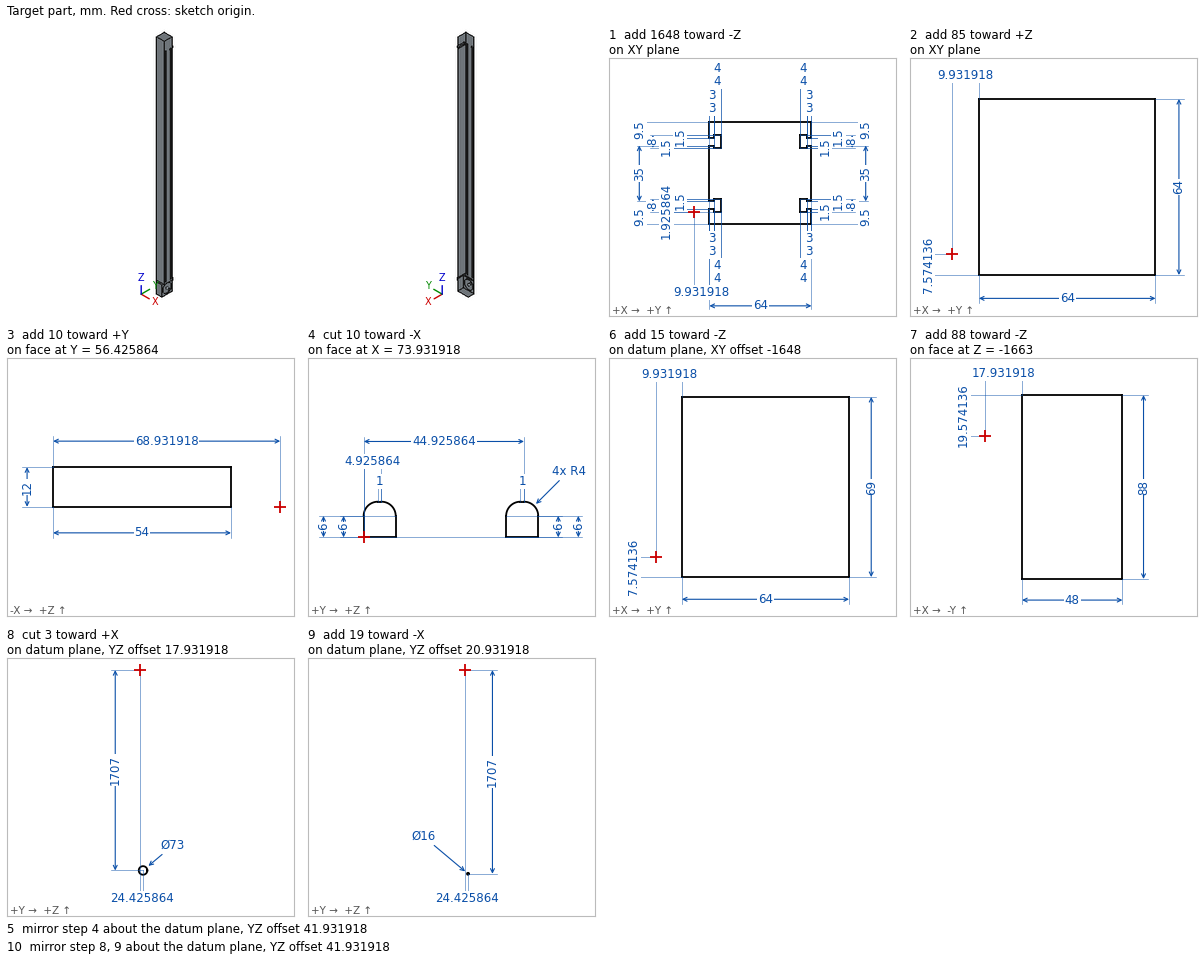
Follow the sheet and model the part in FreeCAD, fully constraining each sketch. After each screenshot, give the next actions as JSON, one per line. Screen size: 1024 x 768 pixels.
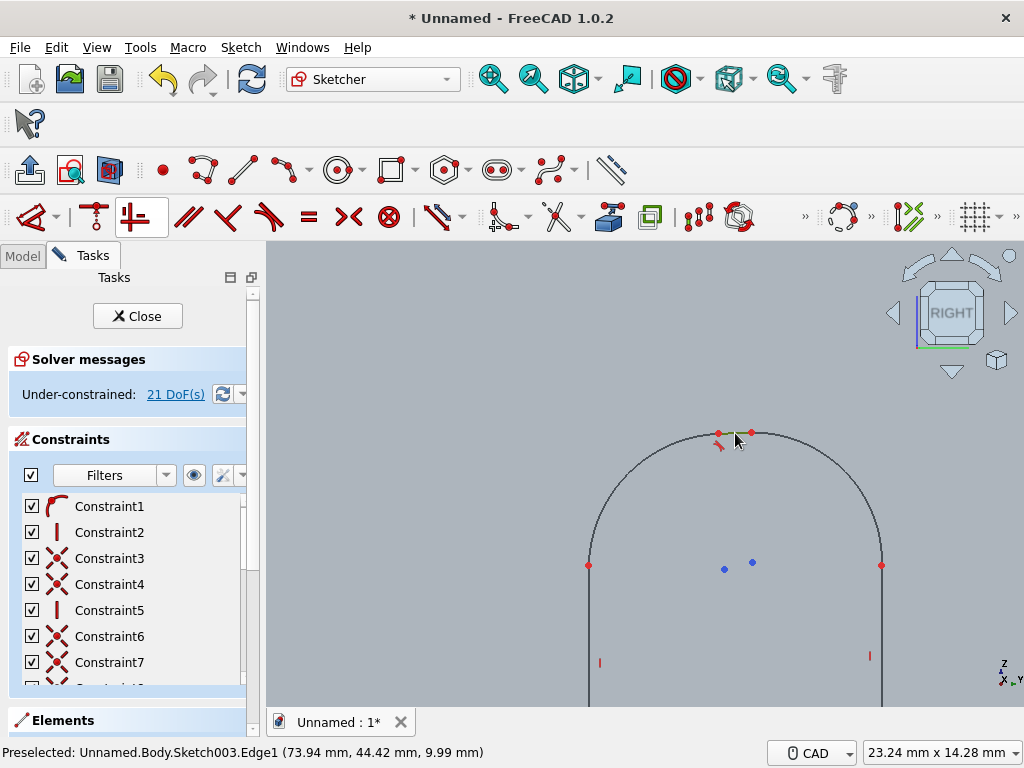
{"action": "scroll", "coordinate": [738, 434], "scroll_direction": "down", "scroll_amount": 7}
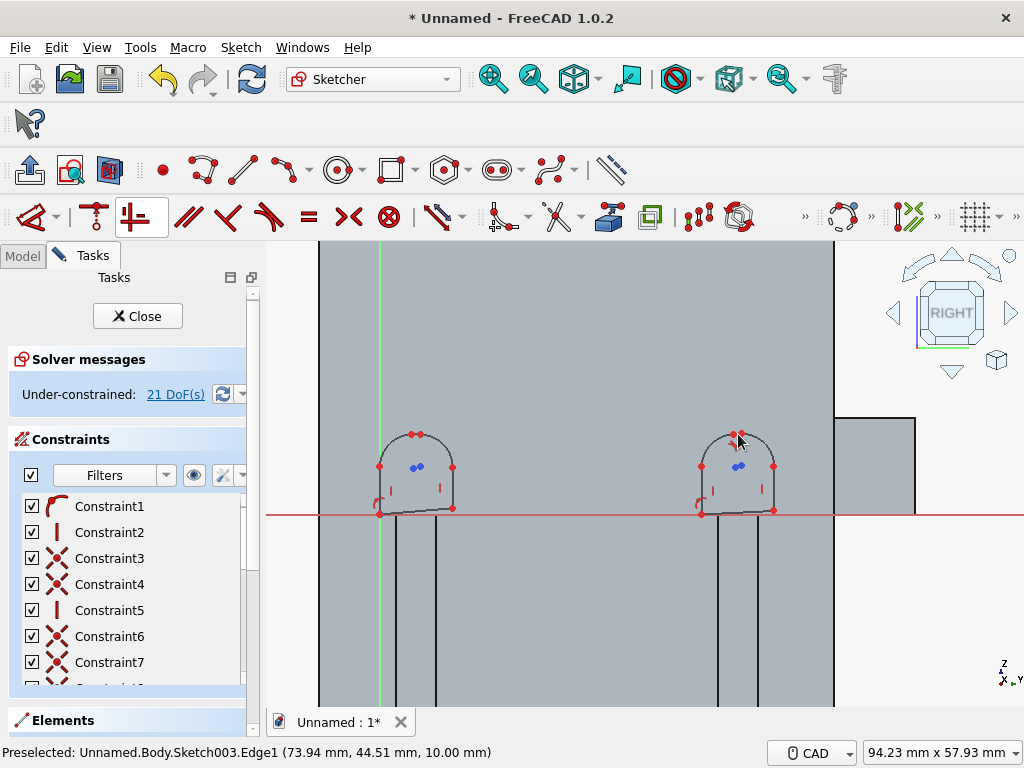
{"action": "left_click", "coordinate": [757, 437]}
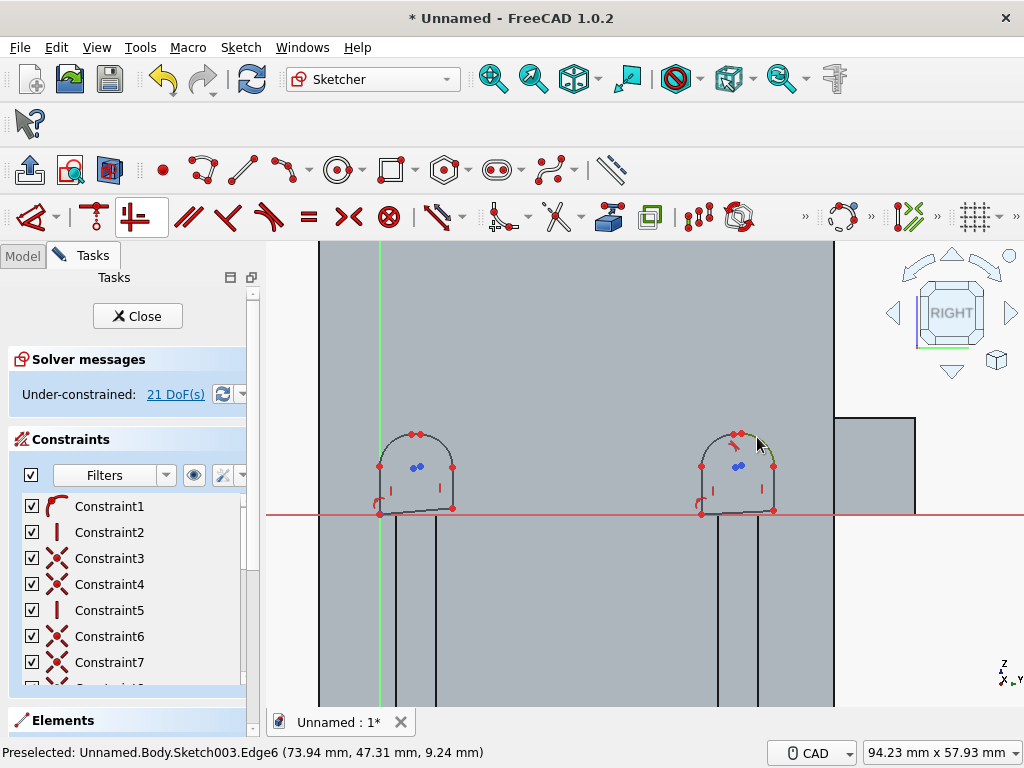
{"action": "left_click", "coordinate": [270, 218]}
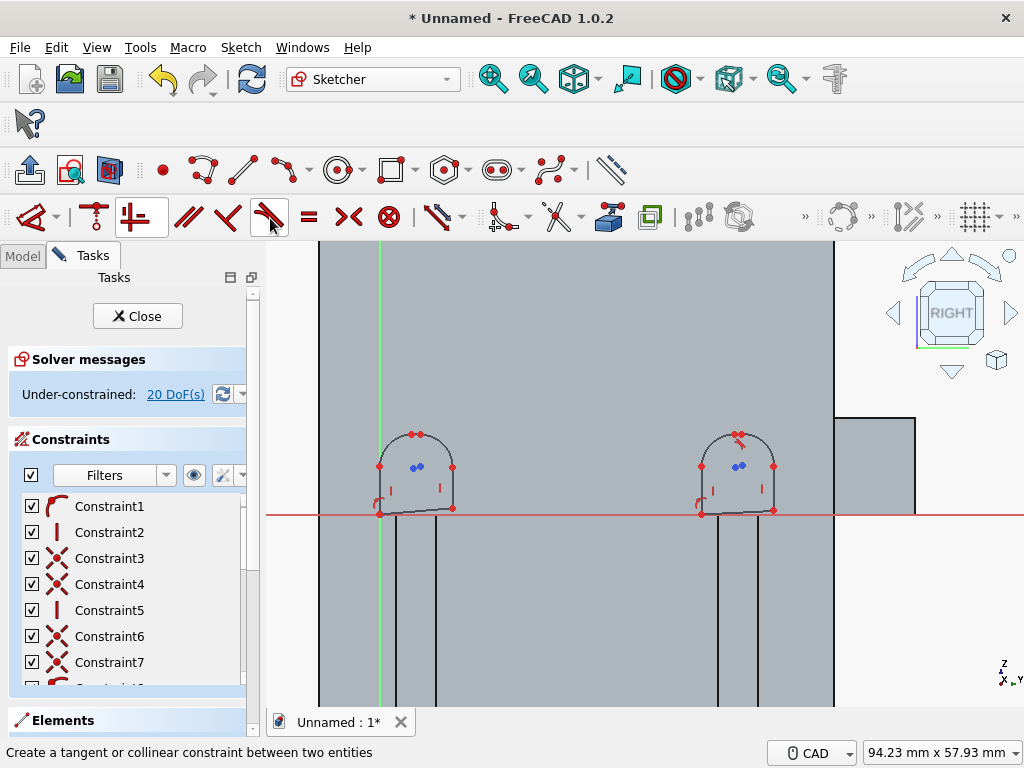
{"action": "left_click", "coordinate": [702, 481]}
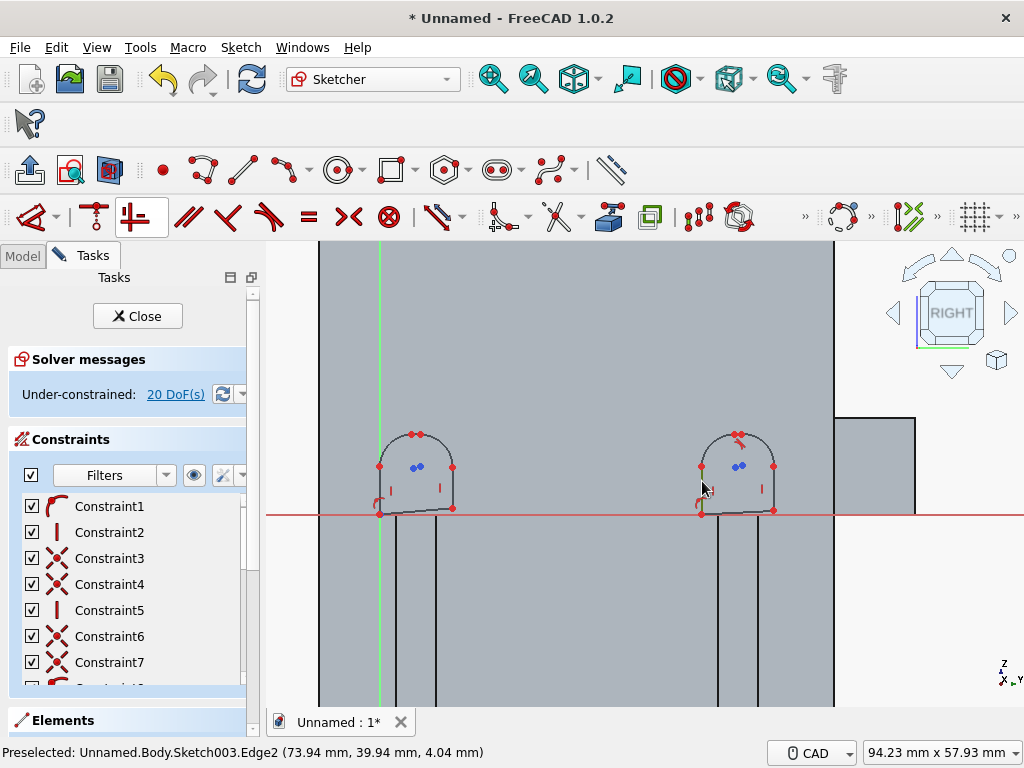
{"action": "left_click", "coordinate": [720, 438]}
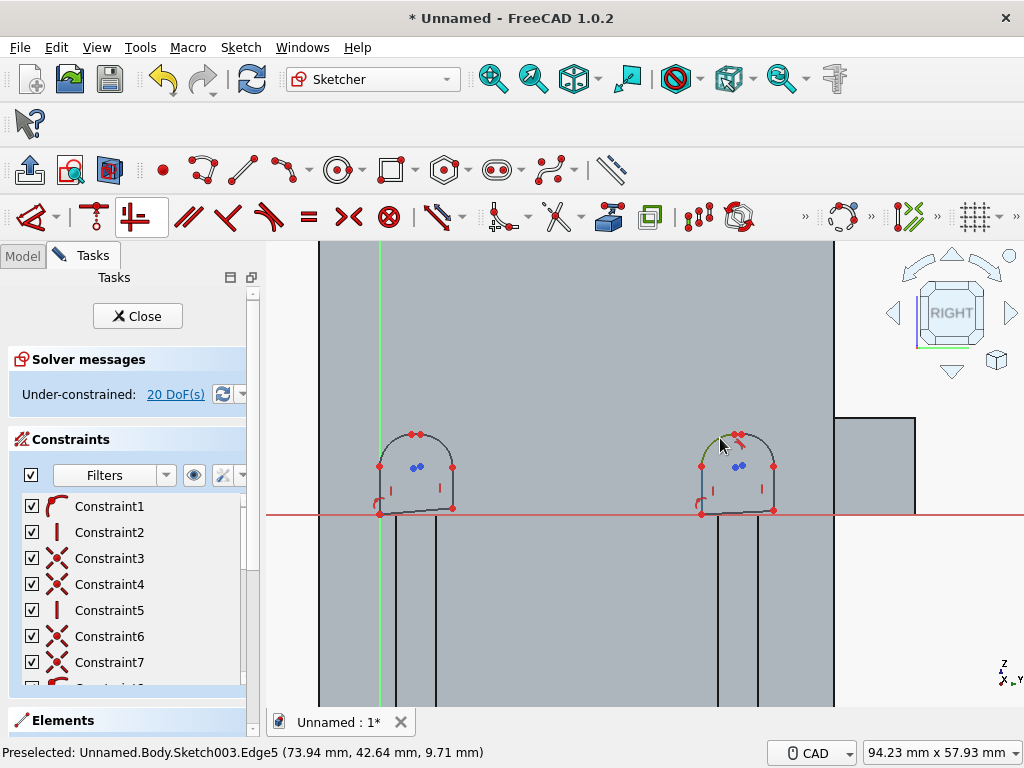
{"action": "left_click", "coordinate": [270, 218]}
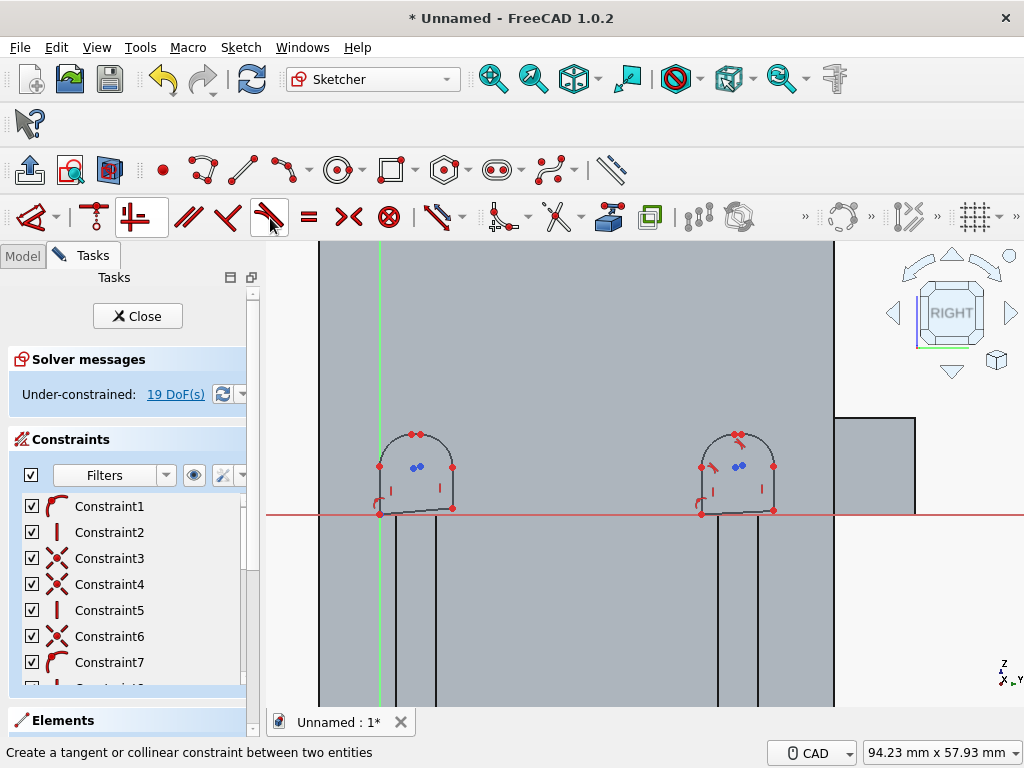
{"action": "left_click", "coordinate": [774, 498]}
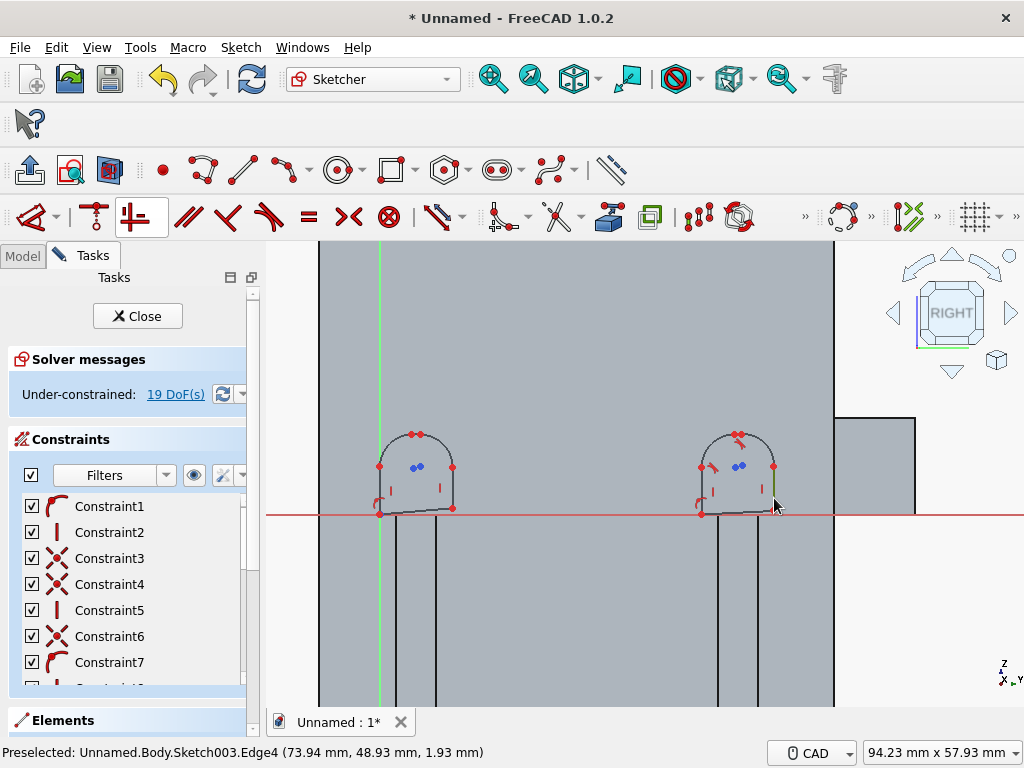
{"action": "left_click", "coordinate": [771, 452]}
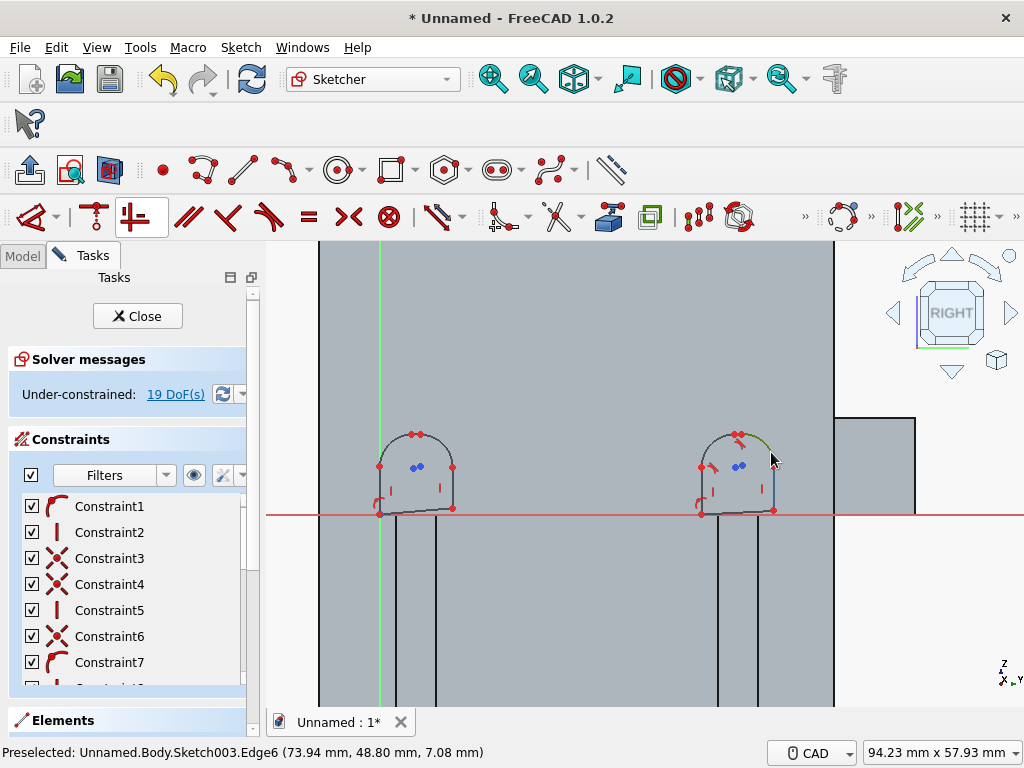
{"action": "left_click", "coordinate": [270, 218]}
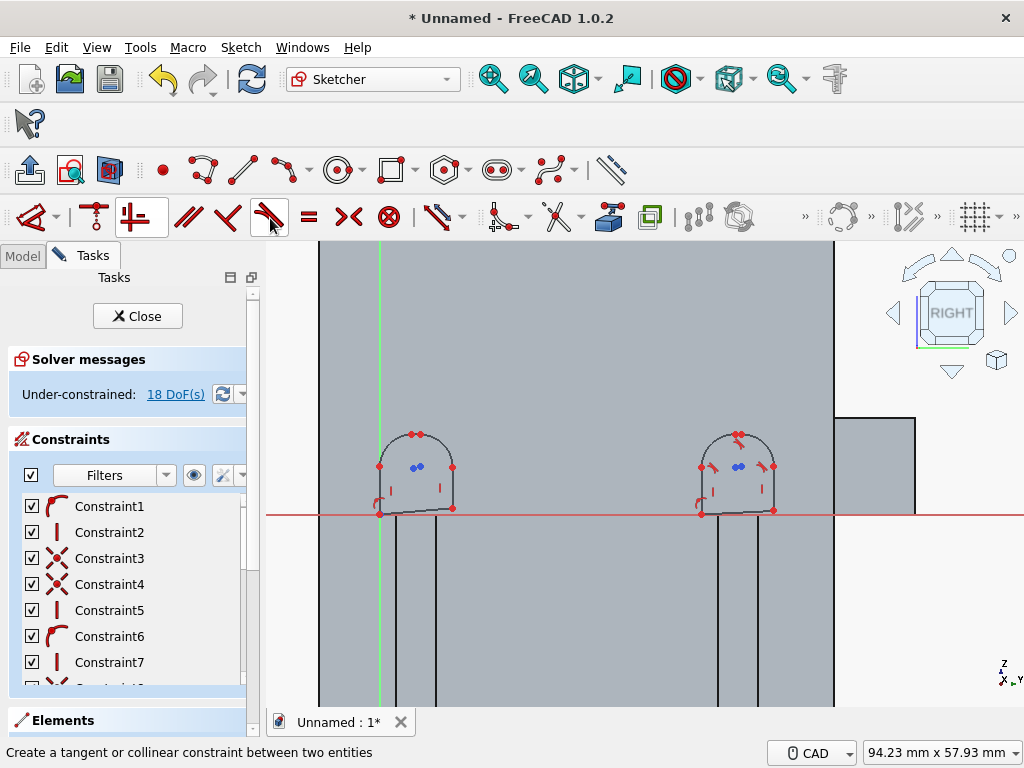
{"action": "scroll", "coordinate": [416, 434], "scroll_direction": "up", "scroll_amount": 6}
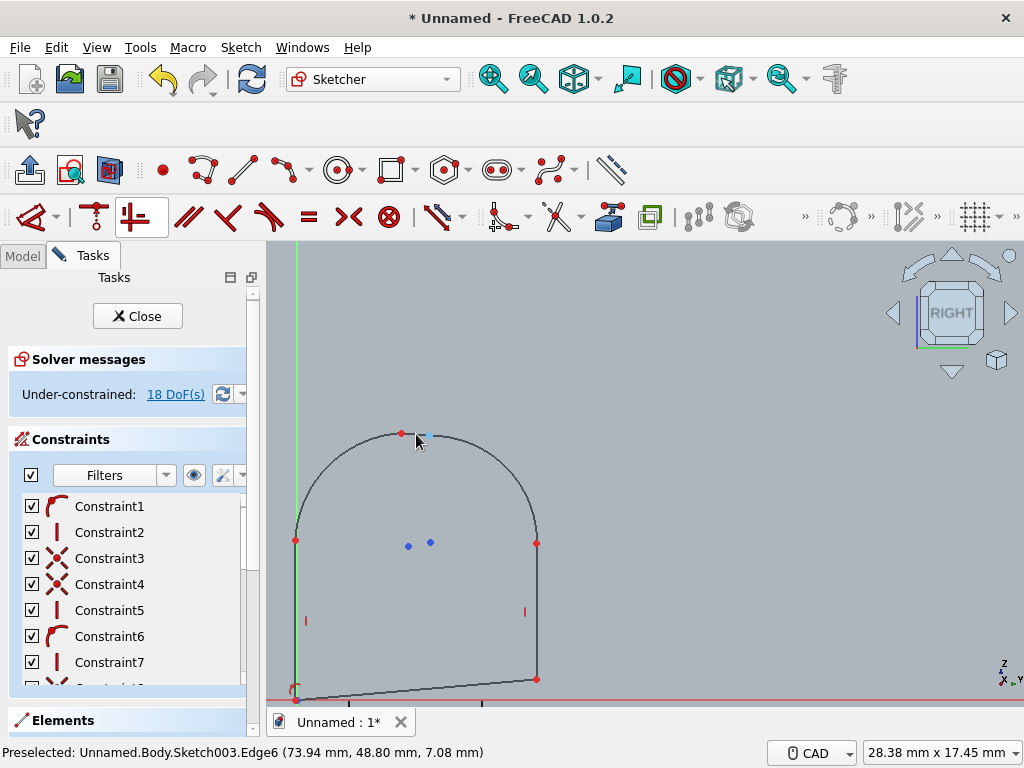
{"action": "left_click", "coordinate": [415, 434]}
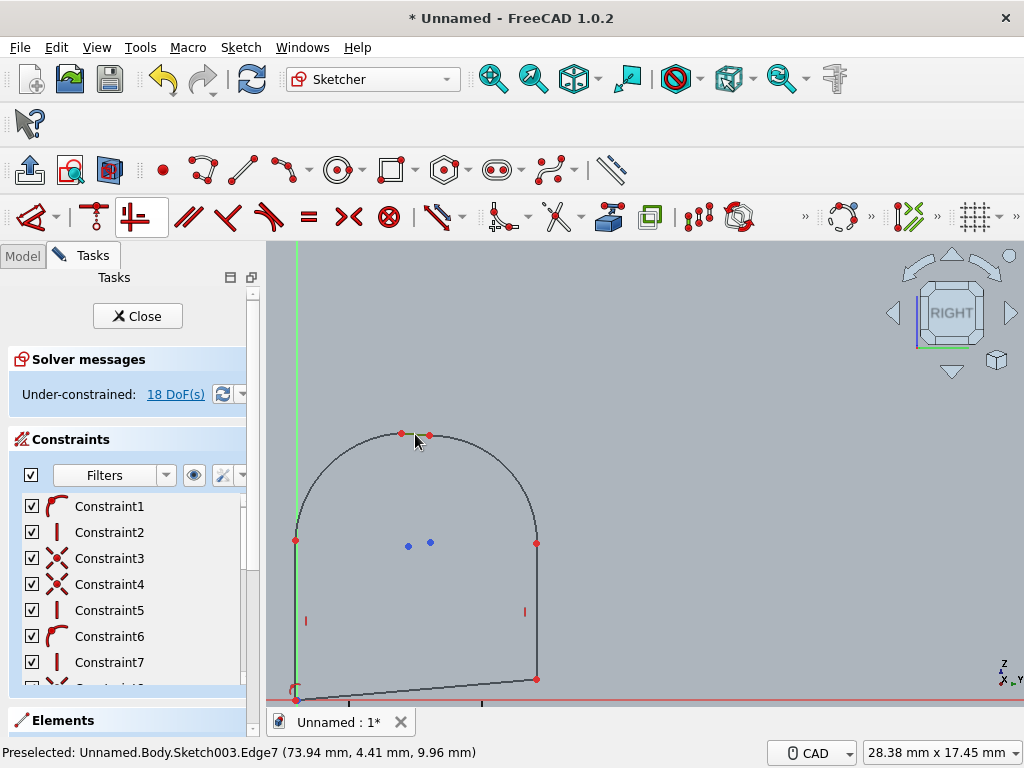
{"action": "left_click", "coordinate": [354, 447]}